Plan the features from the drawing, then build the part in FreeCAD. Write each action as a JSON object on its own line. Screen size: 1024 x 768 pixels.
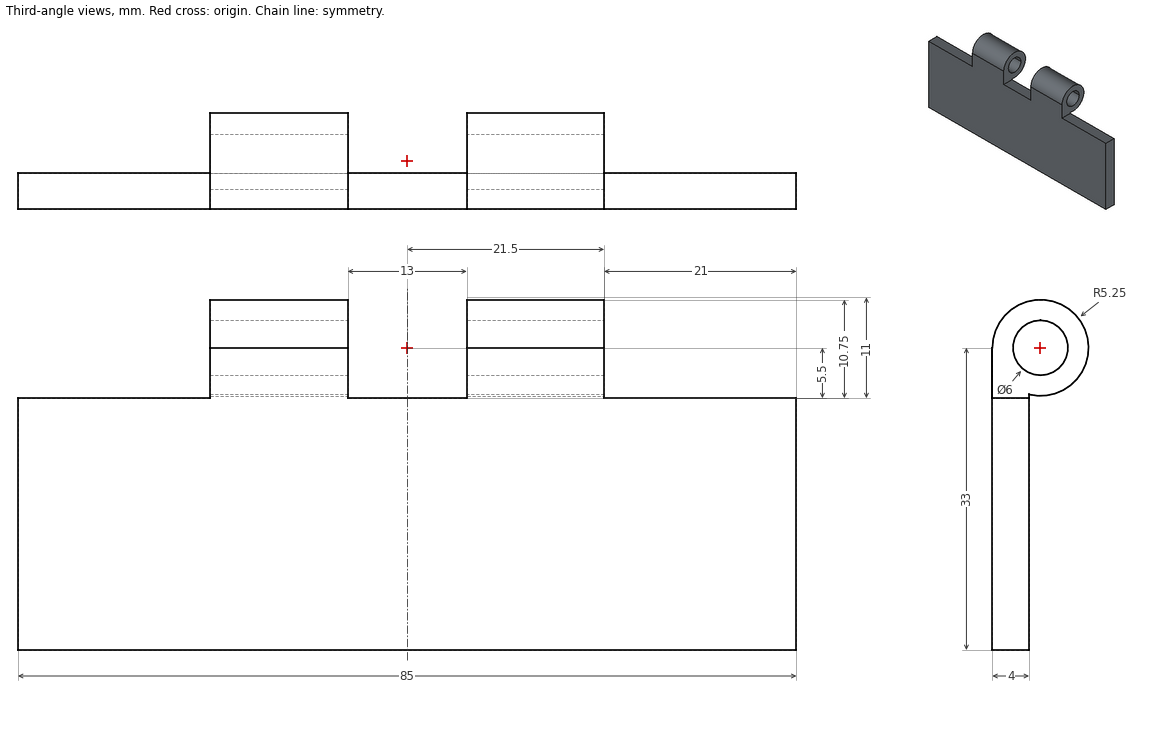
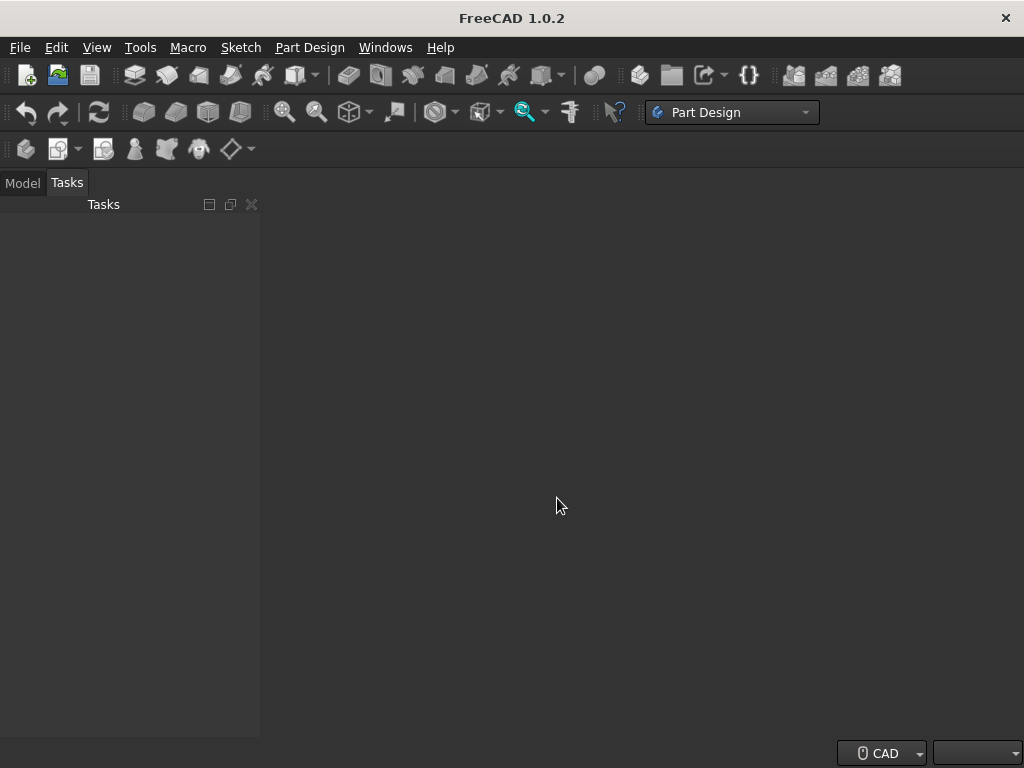
{"action": "left_click", "coordinate": [26, 76]}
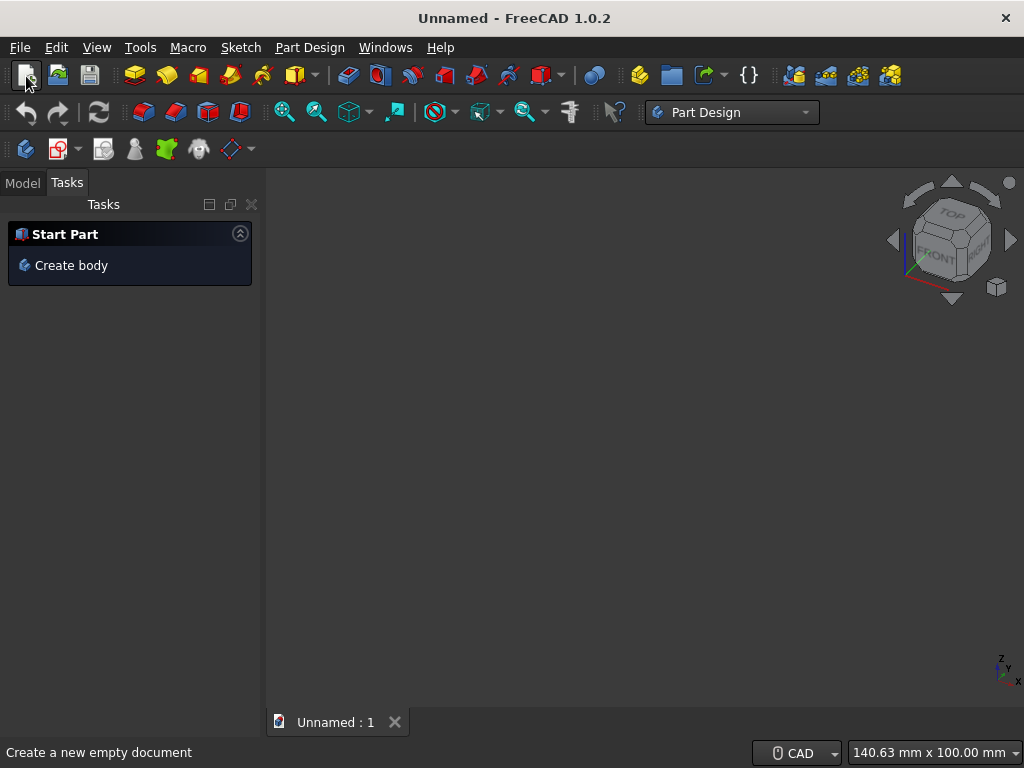
{"action": "left_click", "coordinate": [58, 150]}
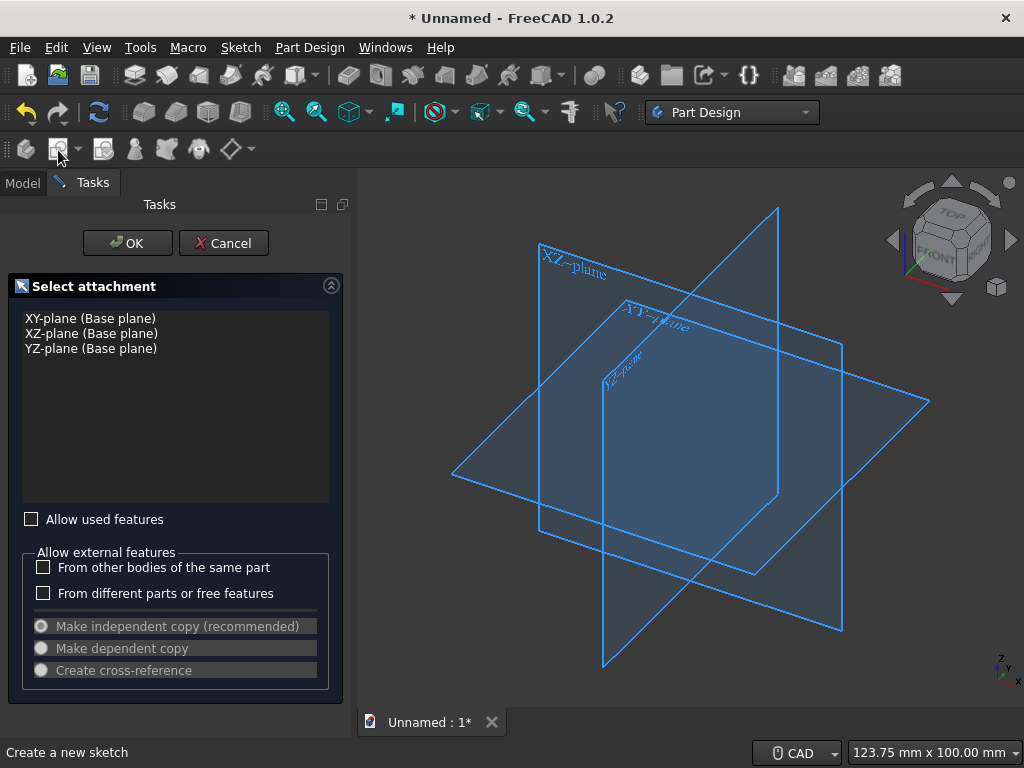
{"action": "left_click", "coordinate": [82, 348]}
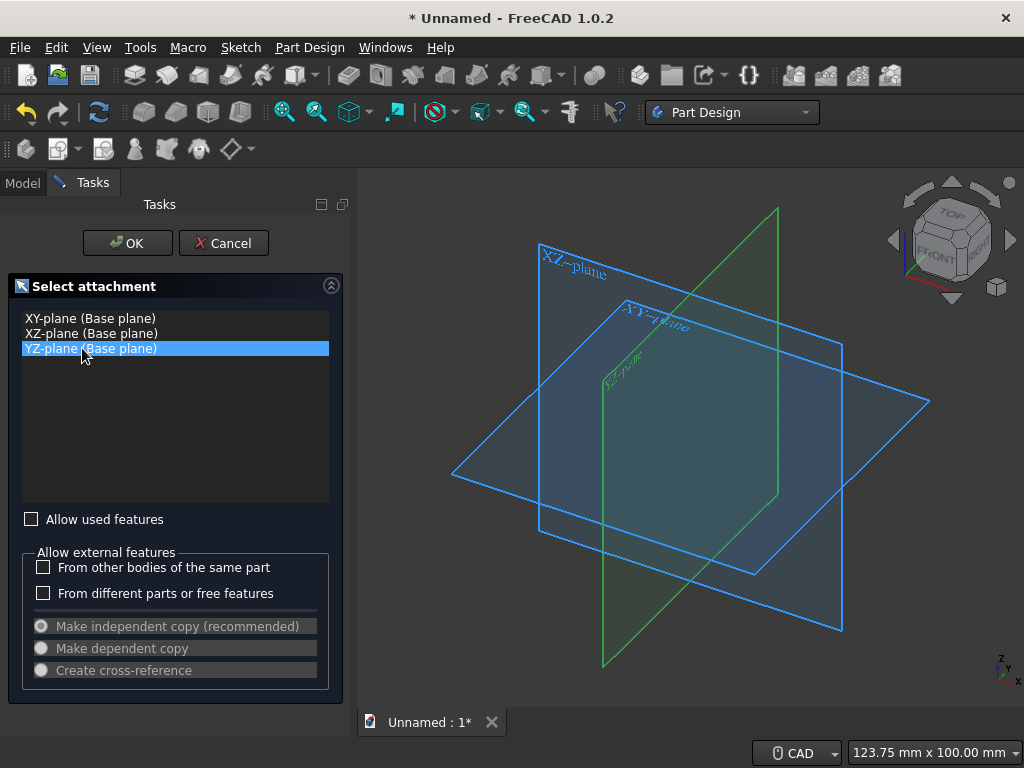
{"action": "left_click", "coordinate": [128, 243]}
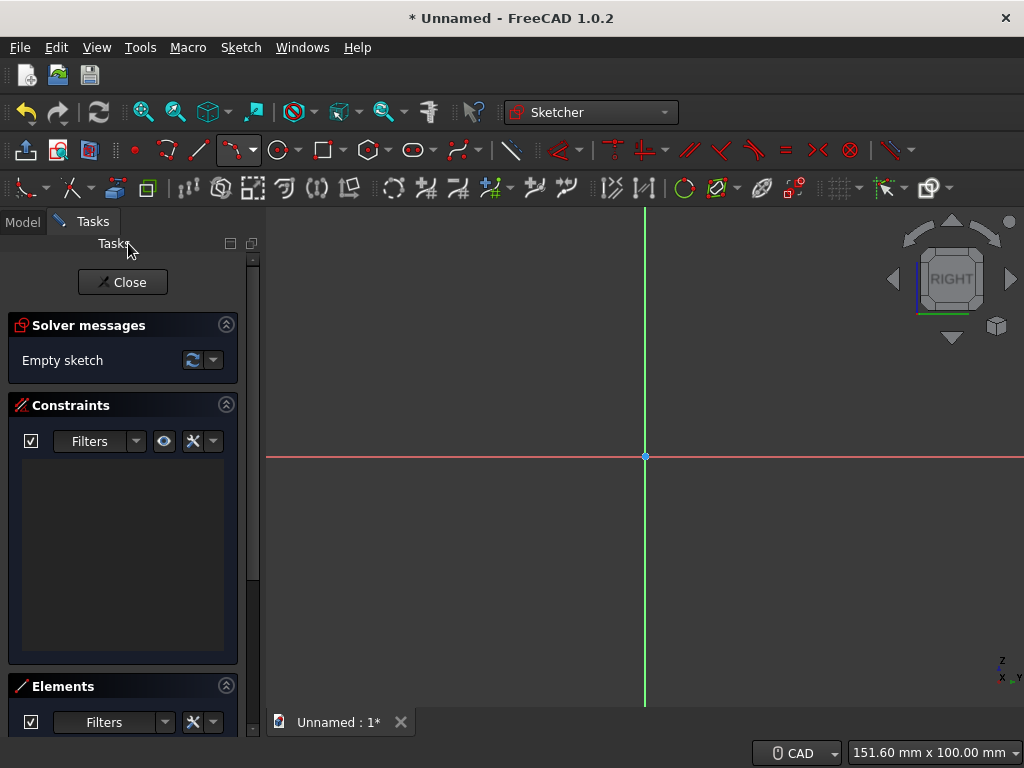
{"action": "scroll", "coordinate": [722, 622], "scroll_direction": "up", "scroll_amount": 3}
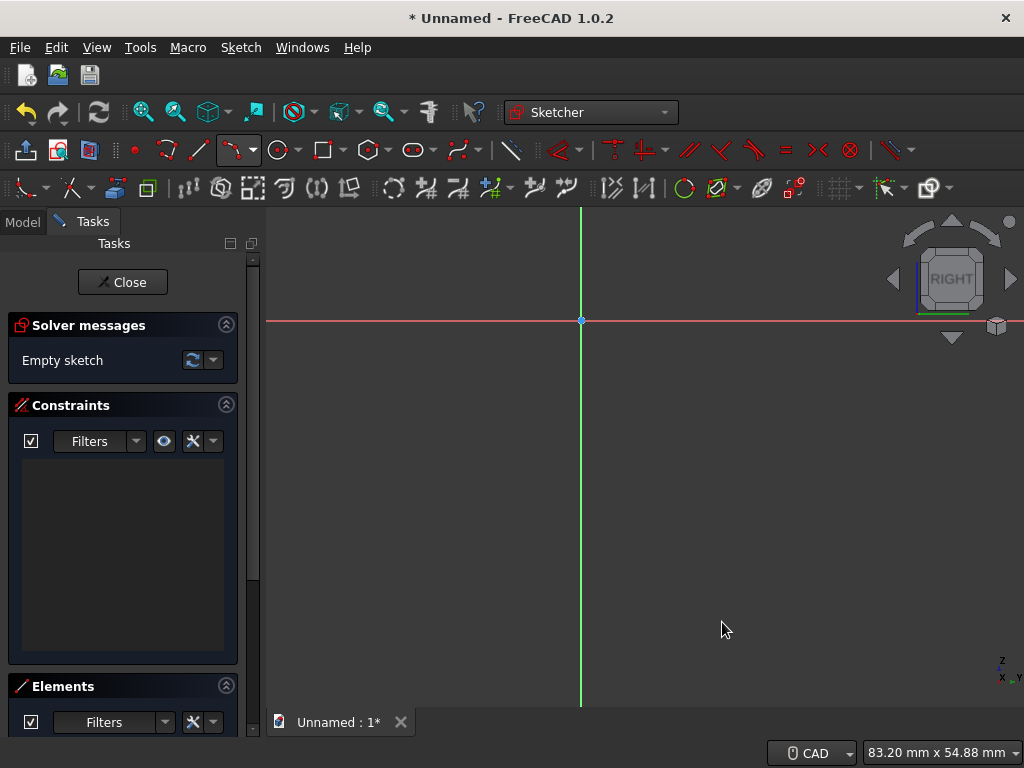
{"action": "left_click", "coordinate": [168, 150]}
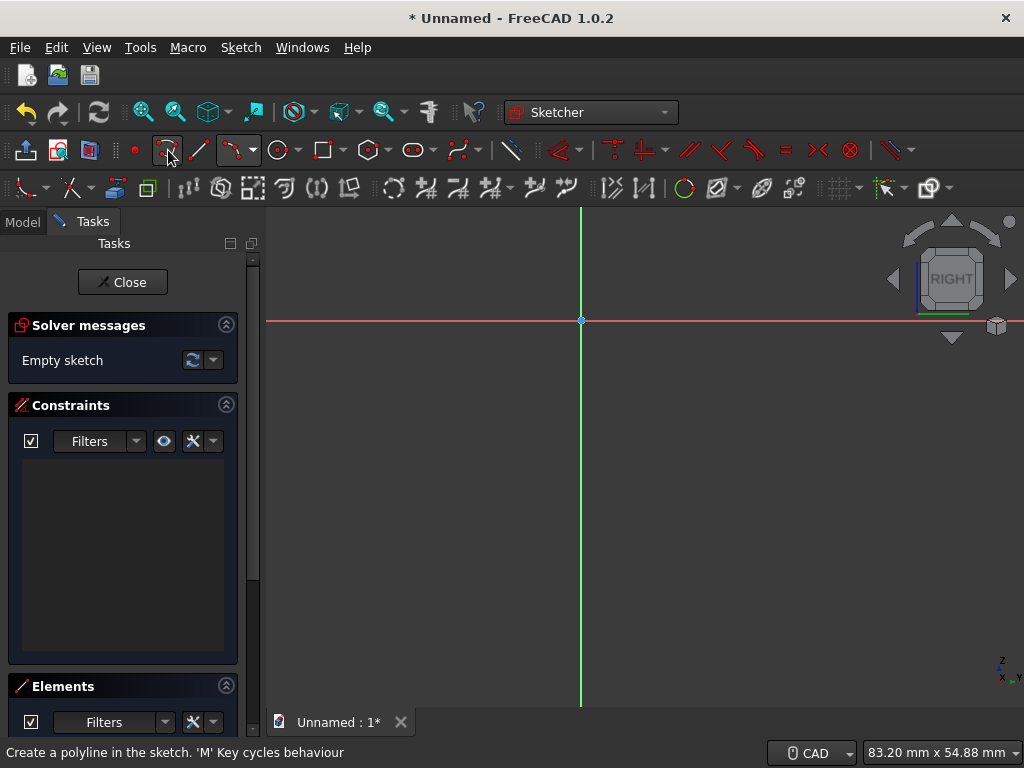
{"action": "left_click", "coordinate": [533, 321]}
{"action": "left_click", "coordinate": [533, 621]}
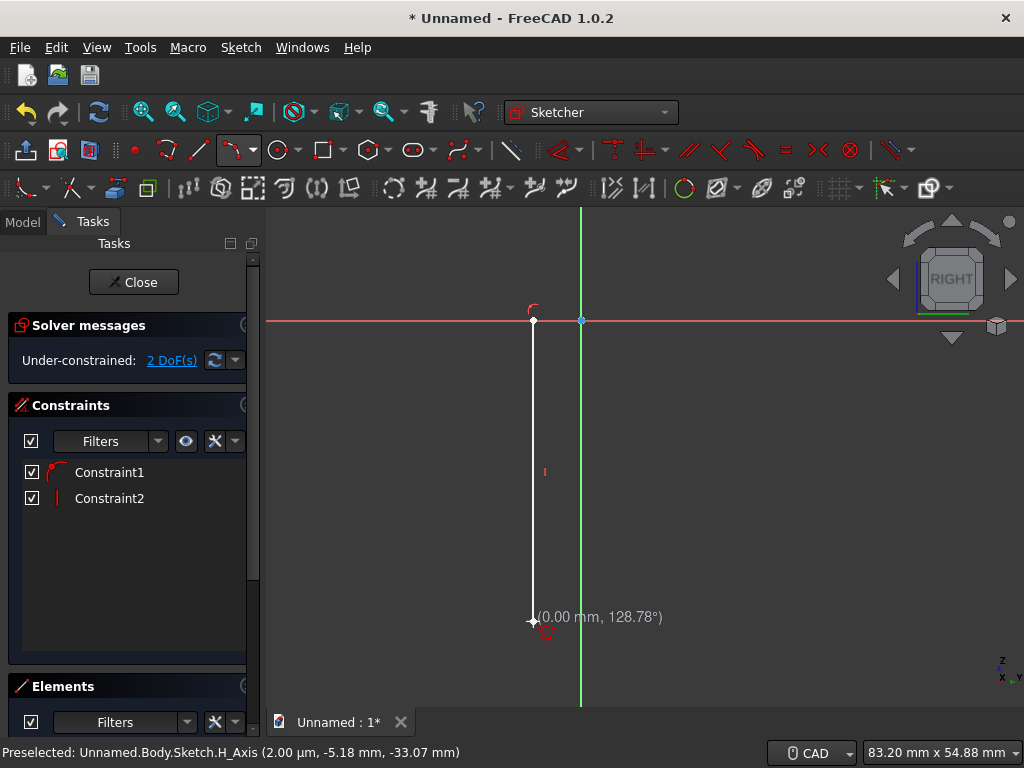
{"action": "scroll", "coordinate": [570, 621], "scroll_direction": "up", "scroll_amount": 2}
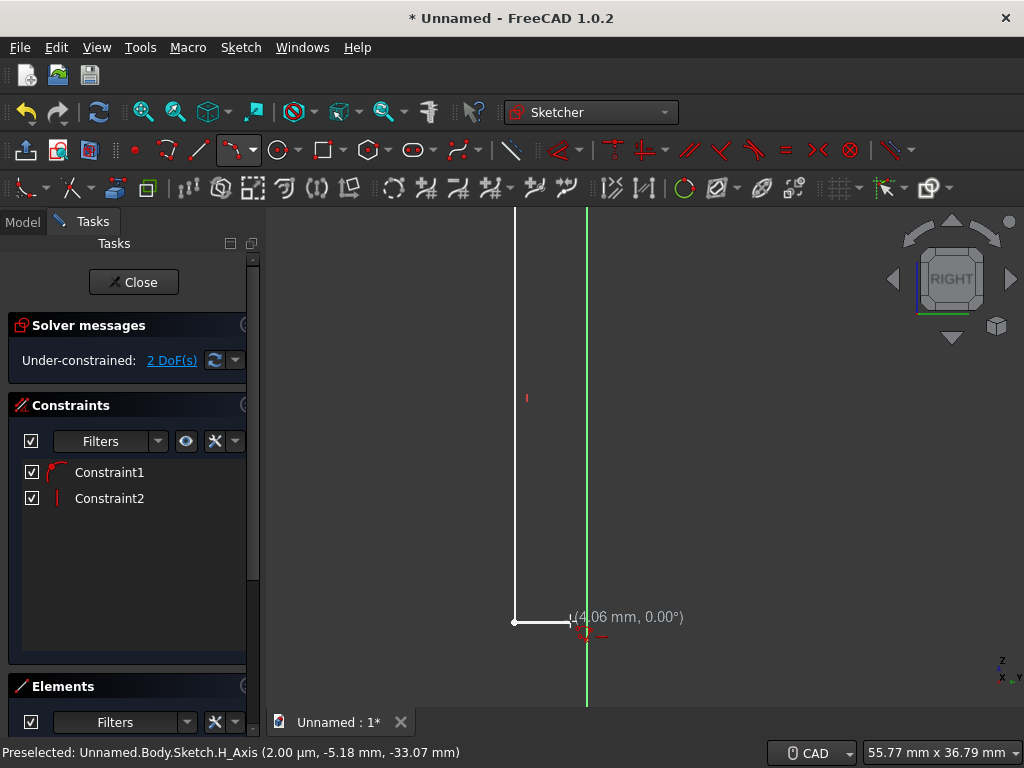
{"action": "left_click", "coordinate": [570, 621]}
{"action": "left_click", "coordinate": [570, 242]}
{"action": "right_click", "coordinate": [570, 242]}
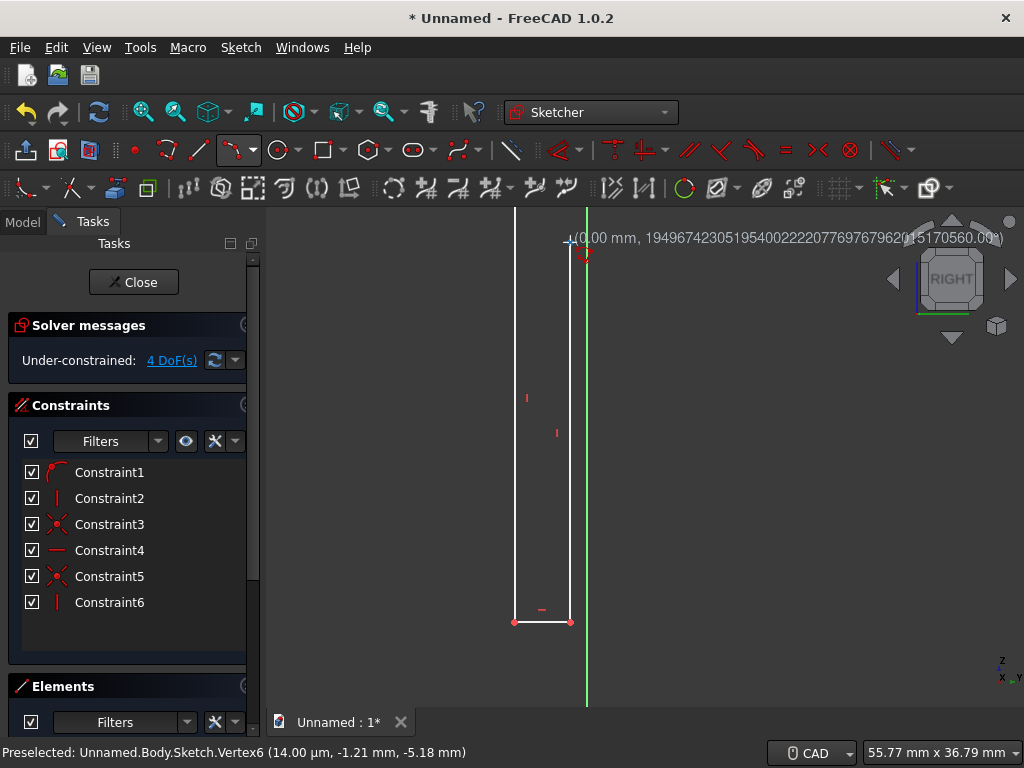
{"action": "left_click", "coordinate": [232, 150]}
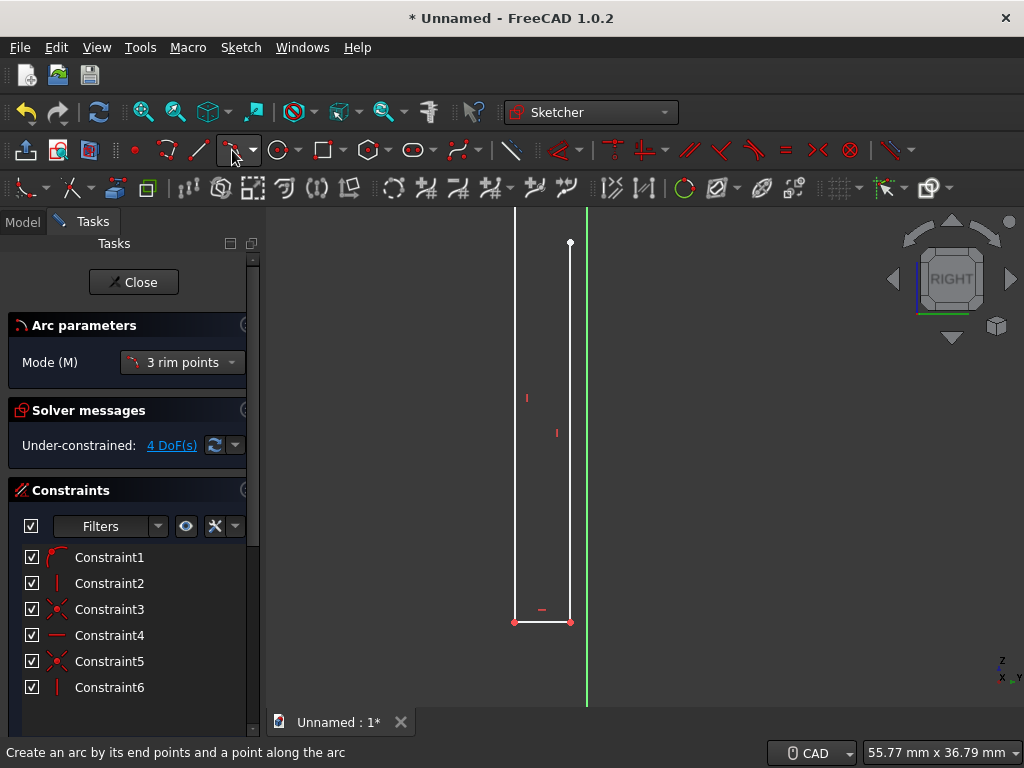
{"action": "left_click", "coordinate": [570, 243]}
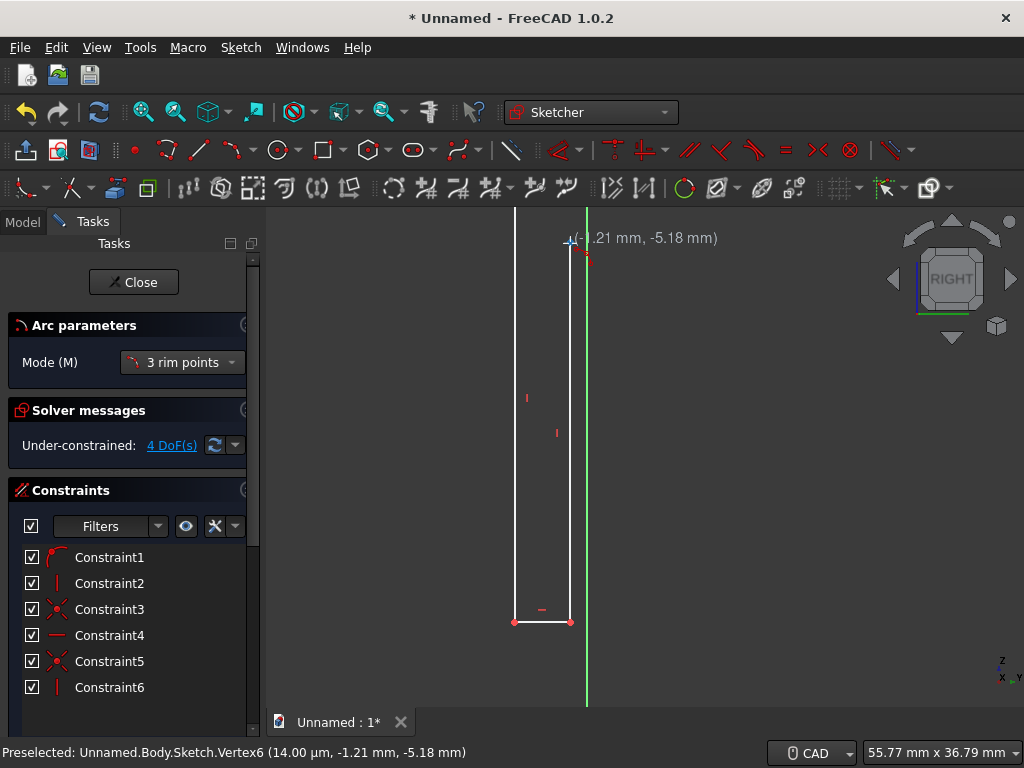
{"action": "scroll", "coordinate": [572, 624], "scroll_direction": "down", "scroll_amount": 2}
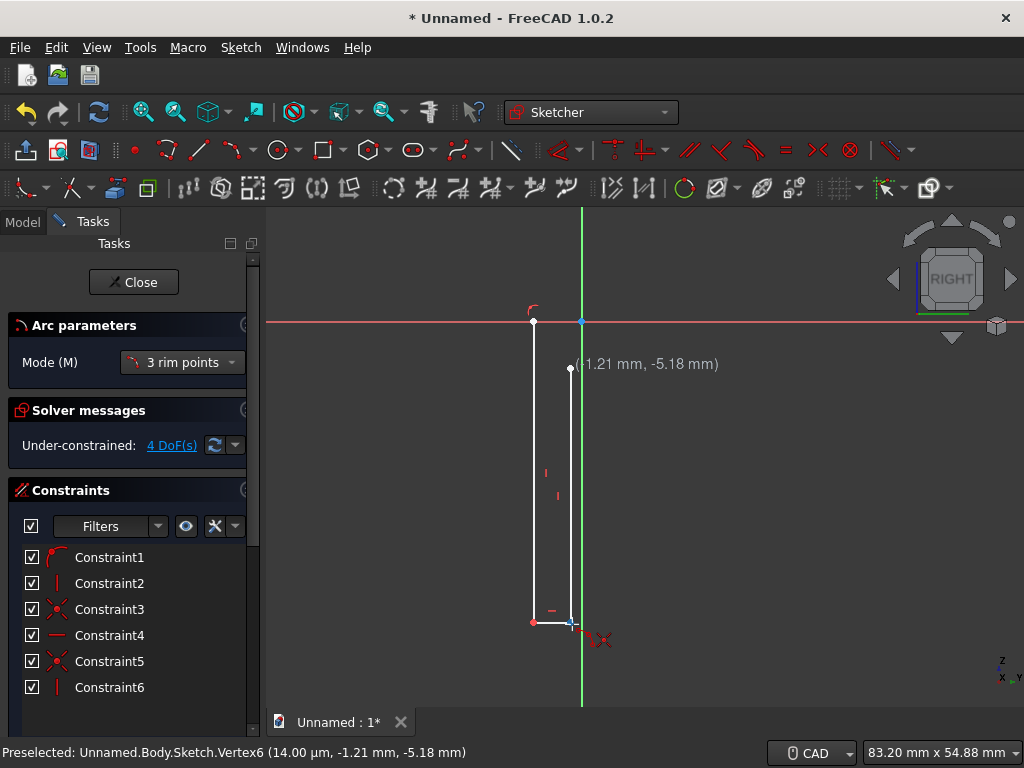
{"action": "left_click", "coordinate": [534, 322]}
{"action": "left_click", "coordinate": [619, 292]}
{"action": "key", "text": "Escape"}